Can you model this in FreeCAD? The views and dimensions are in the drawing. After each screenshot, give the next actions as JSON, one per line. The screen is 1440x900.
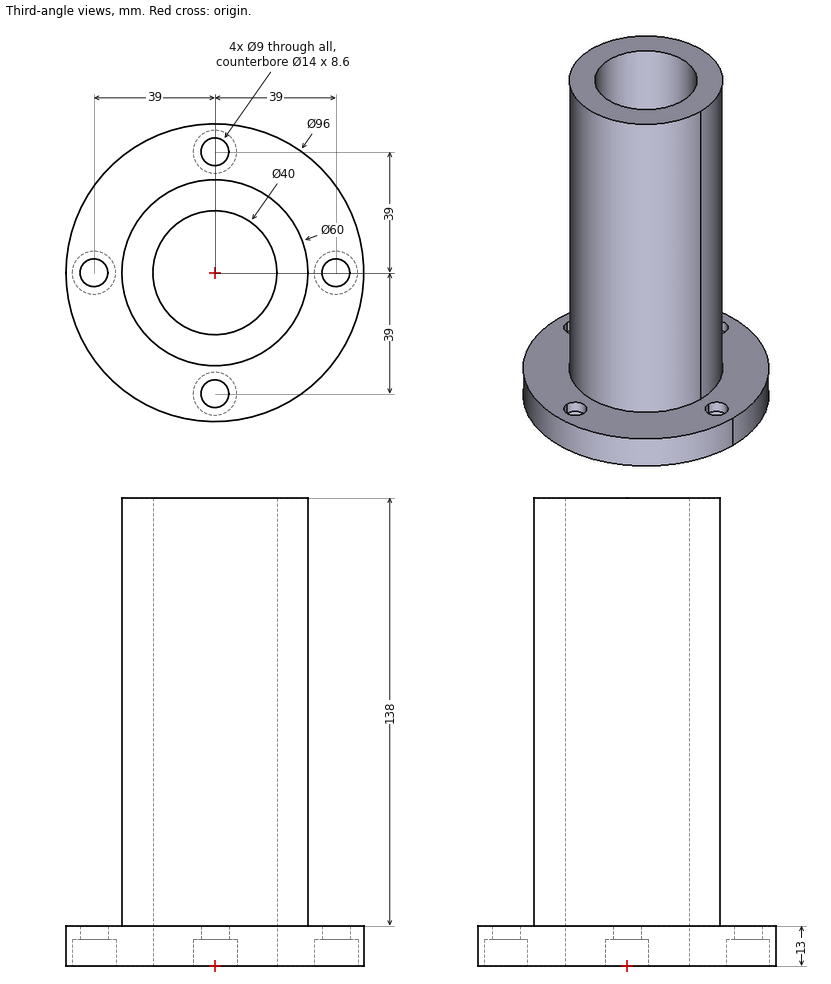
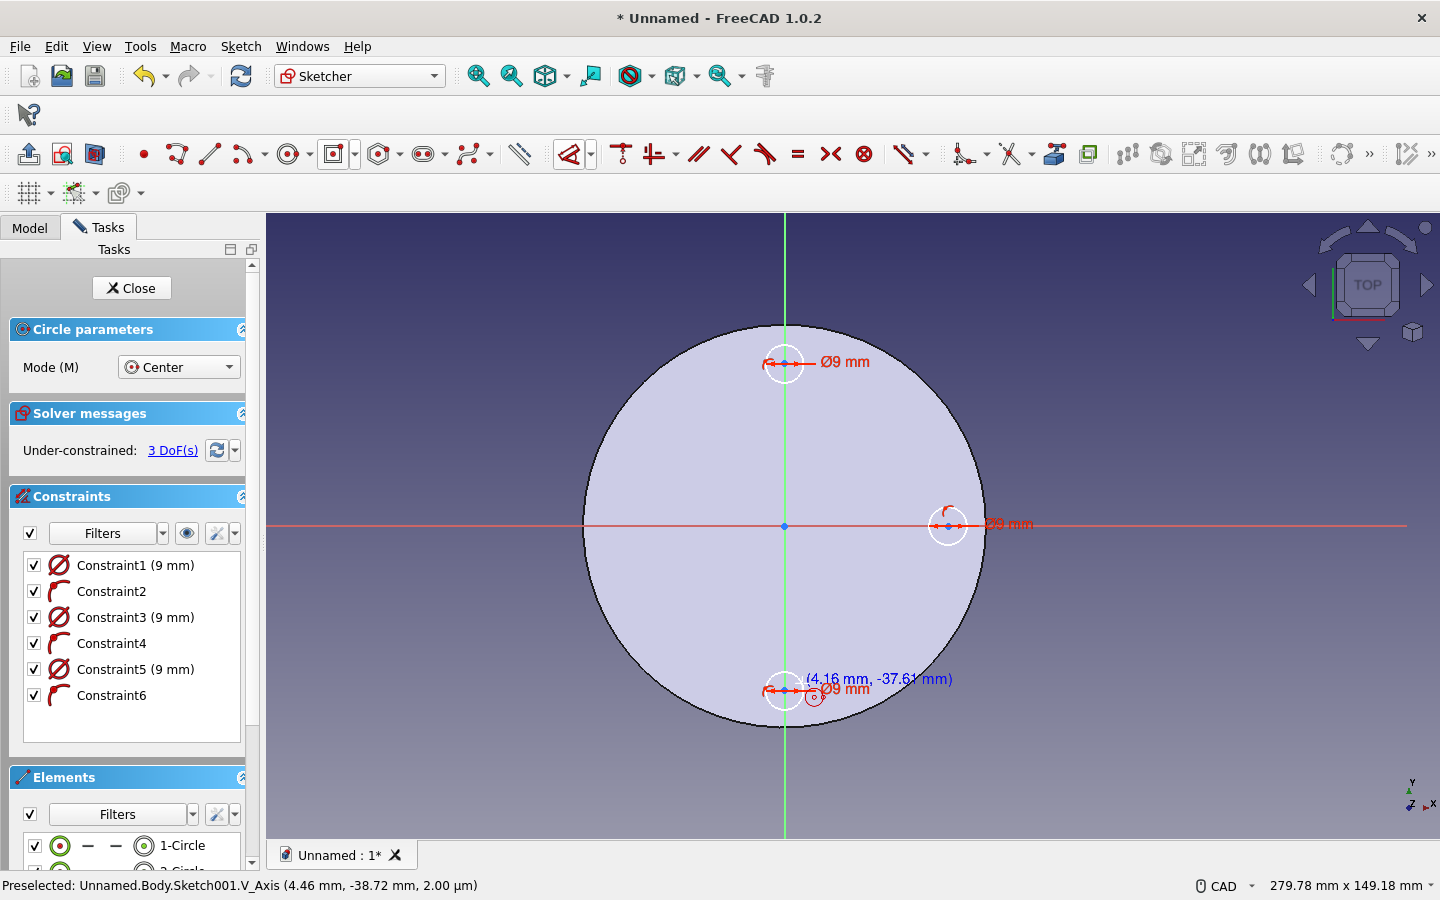
{"action": "left_click", "coordinate": [621, 526]}
{"action": "mouse_move", "coordinate": [627, 508]}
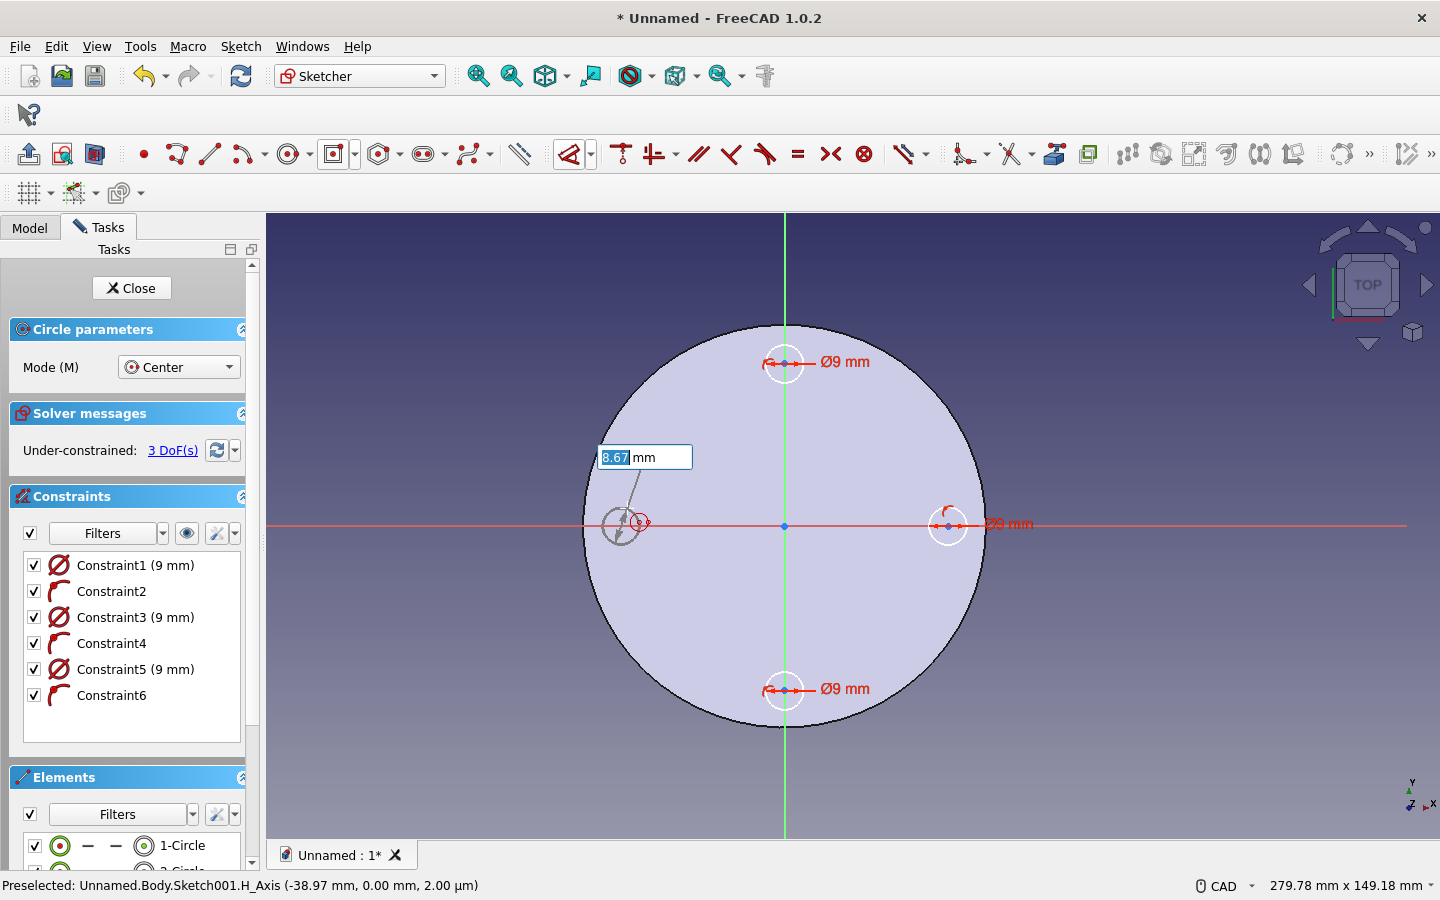
{"action": "type", "text": "9"}
{"action": "key", "text": "Return"}
{"action": "key", "text": "Escape"}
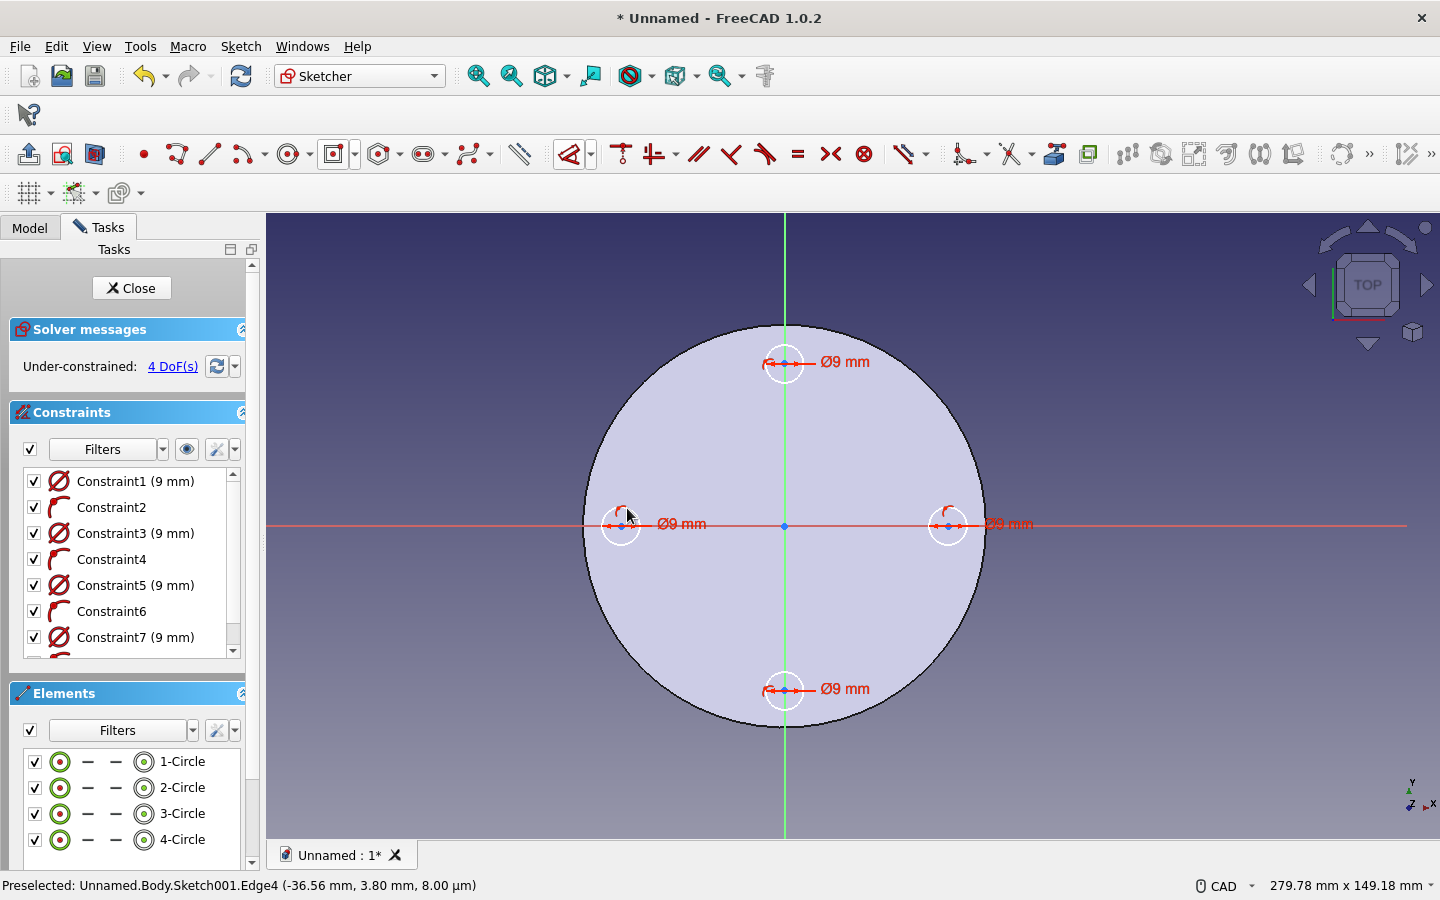
{"action": "left_click", "coordinate": [568, 154]}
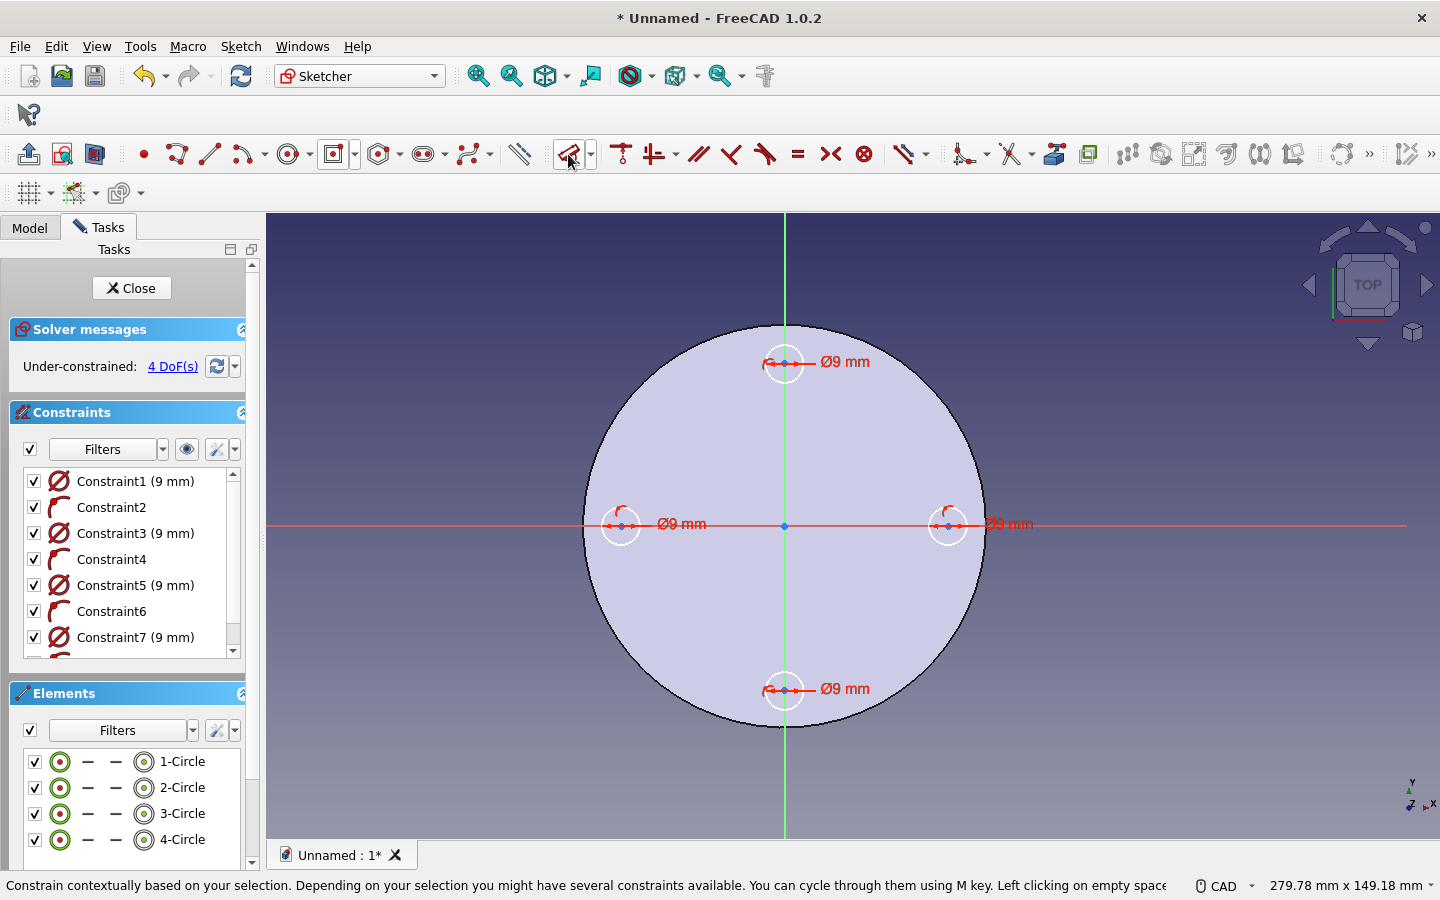
{"action": "left_click", "coordinate": [785, 364]}
{"action": "left_click", "coordinate": [819, 445]}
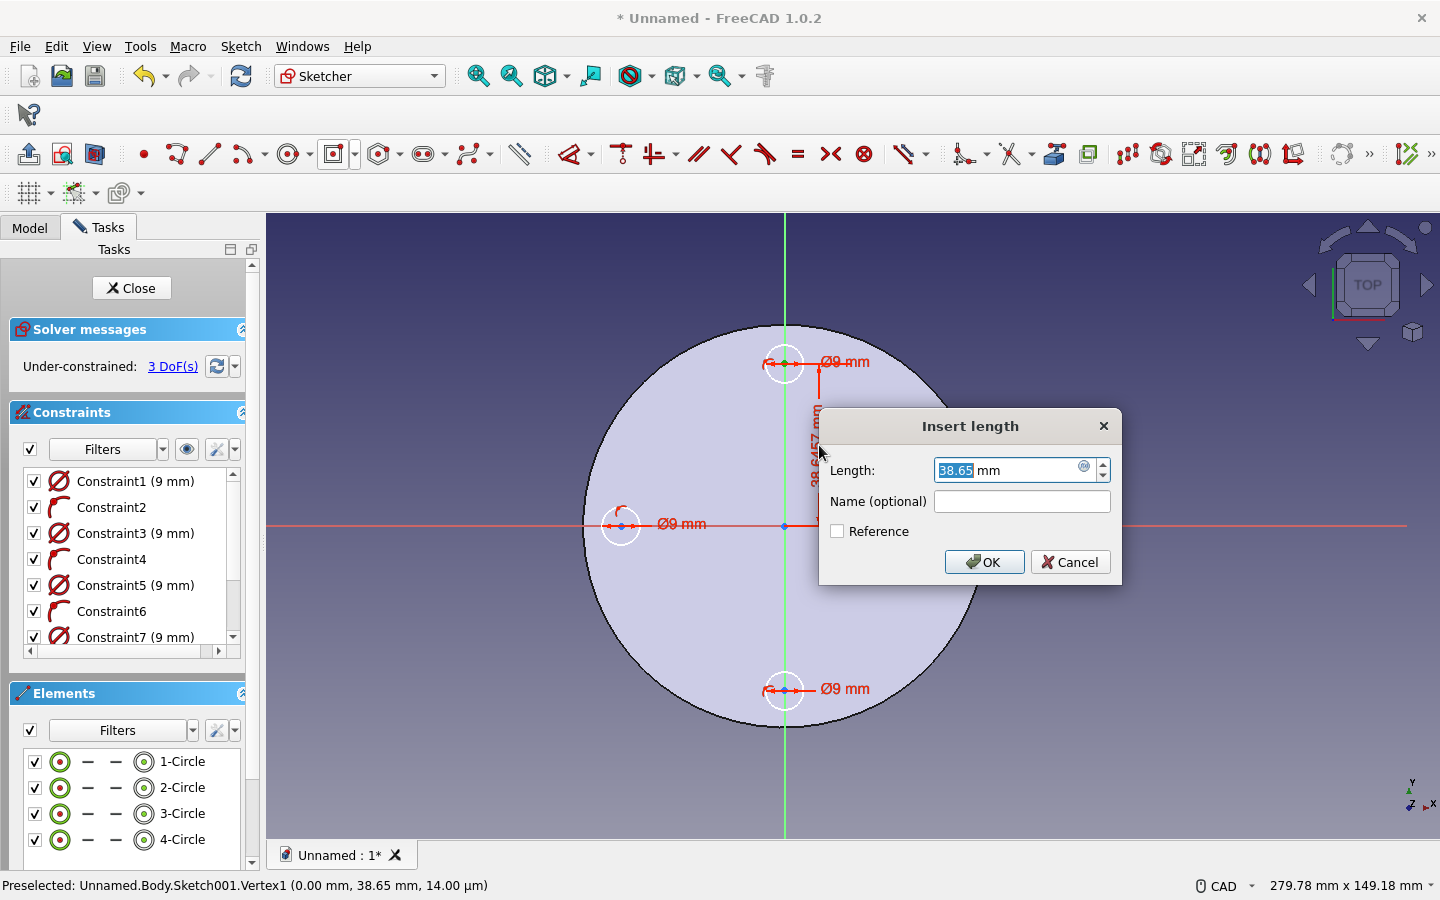
{"action": "type", "text": "39"}
{"action": "key", "text": "Return"}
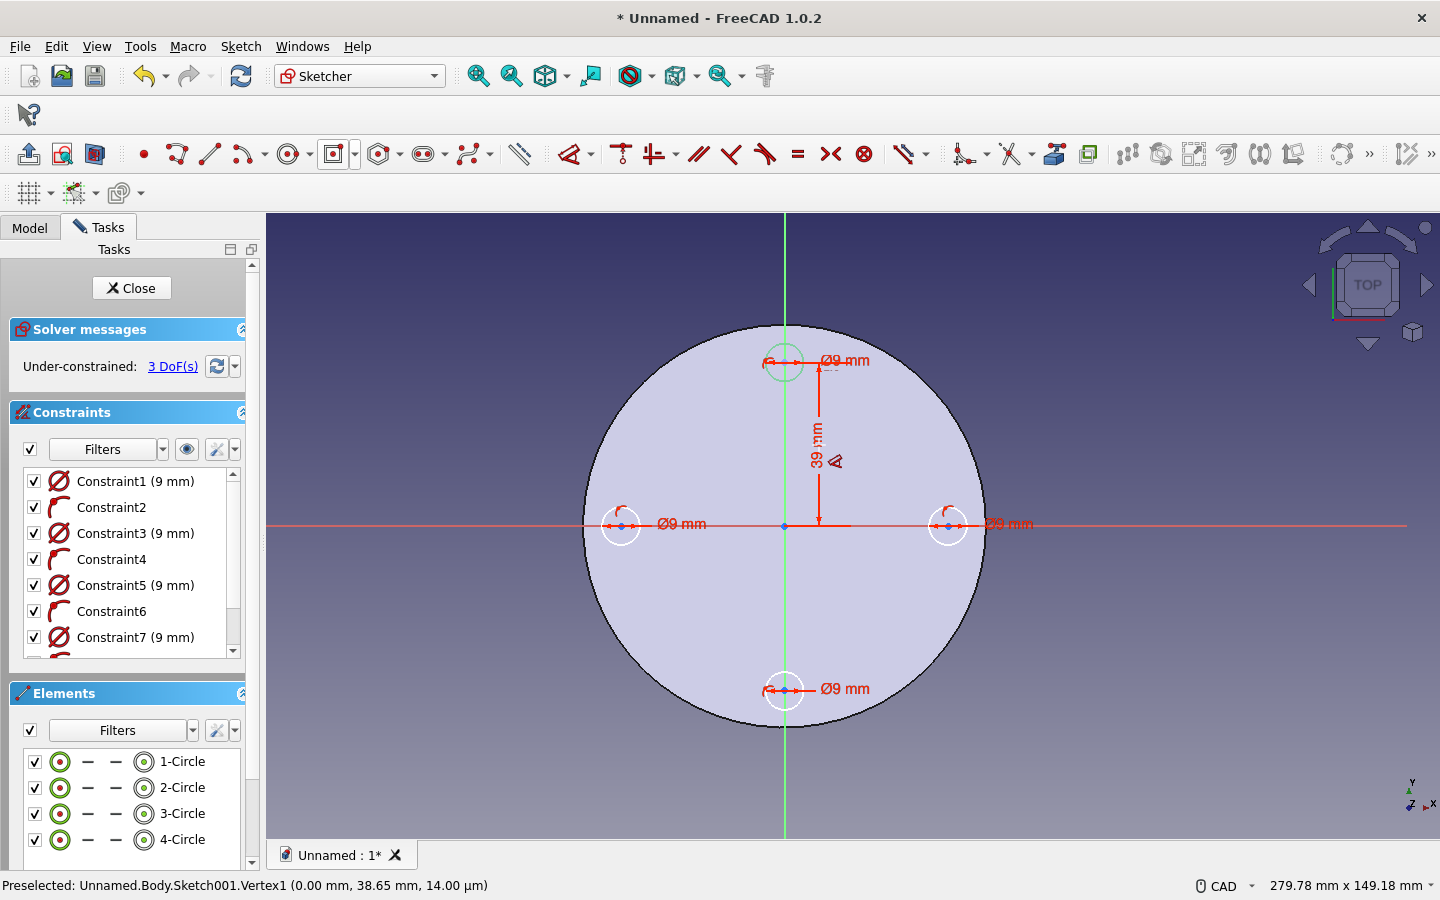
{"action": "left_click", "coordinate": [948, 526]}
{"action": "left_click", "coordinate": [866, 560]}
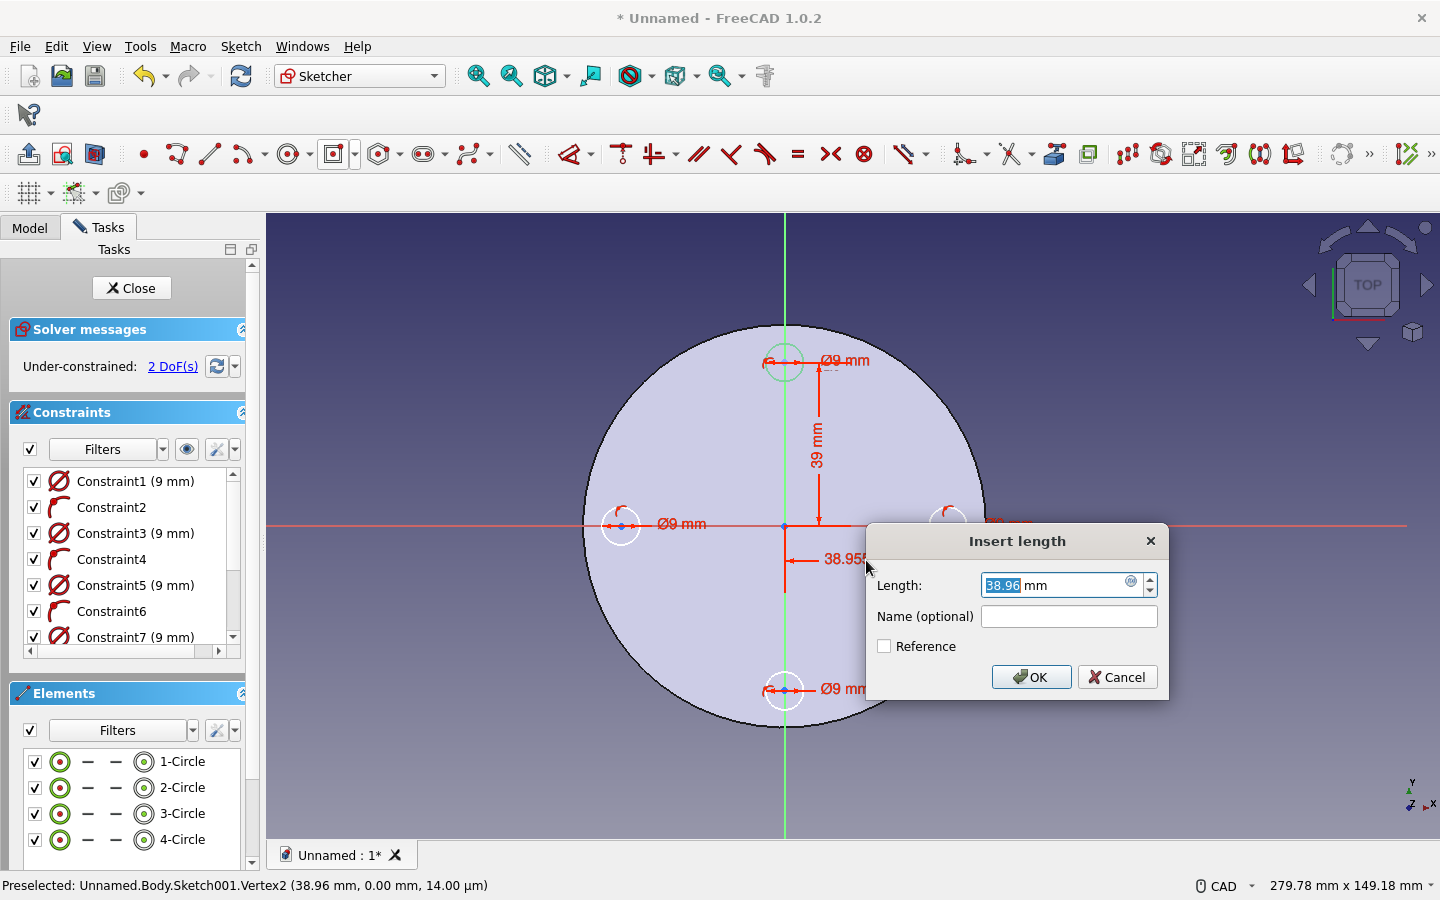
{"action": "type", "text": "39"}
{"action": "key", "text": "Return"}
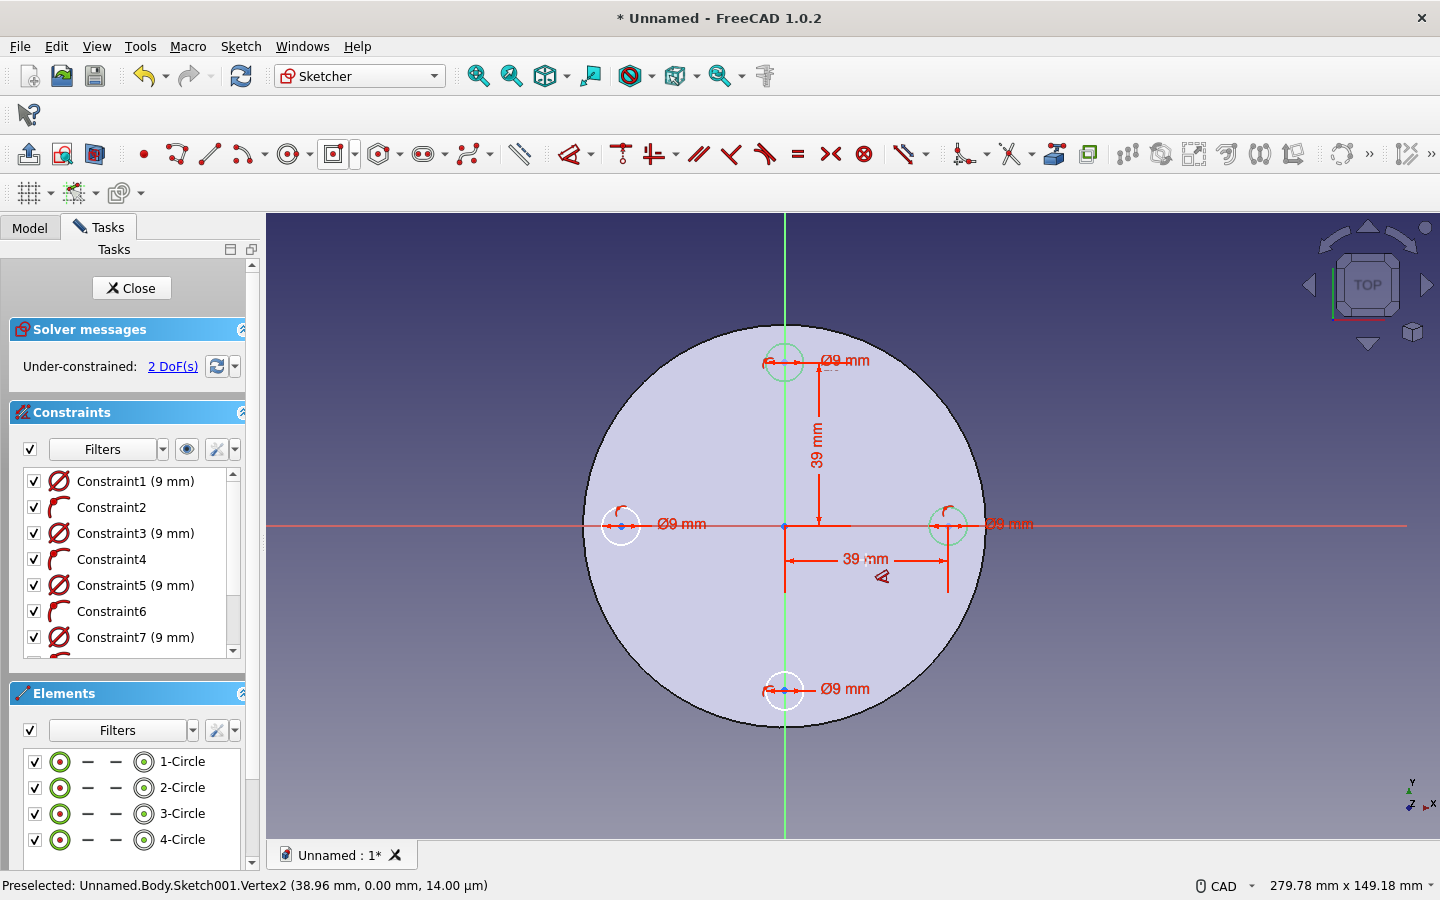
{"action": "left_click", "coordinate": [785, 691]}
{"action": "left_click", "coordinate": [819, 609]}